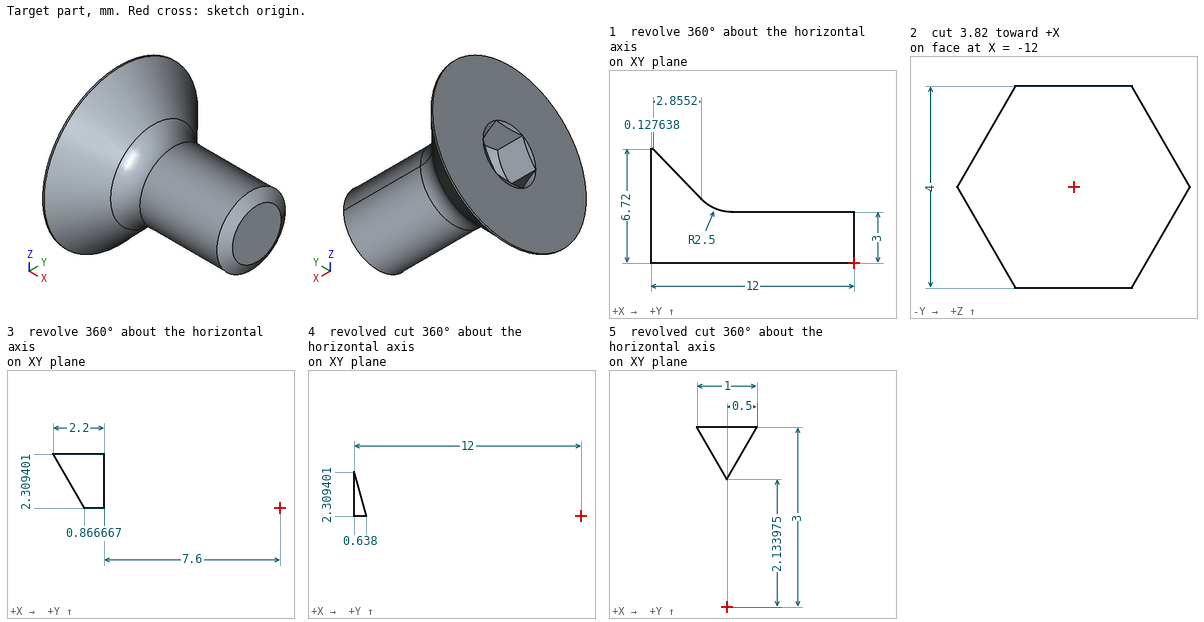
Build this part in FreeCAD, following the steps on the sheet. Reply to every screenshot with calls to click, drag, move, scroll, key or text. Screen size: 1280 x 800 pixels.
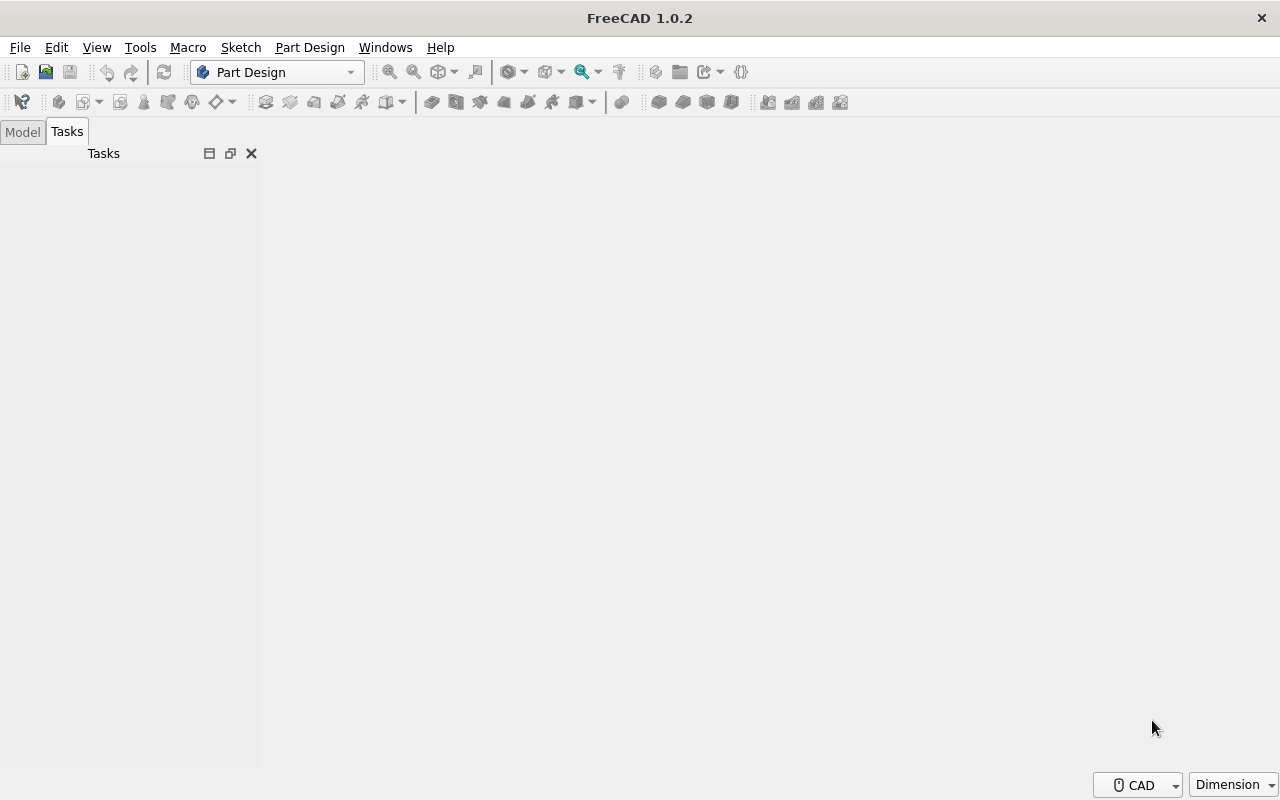
click(22, 72)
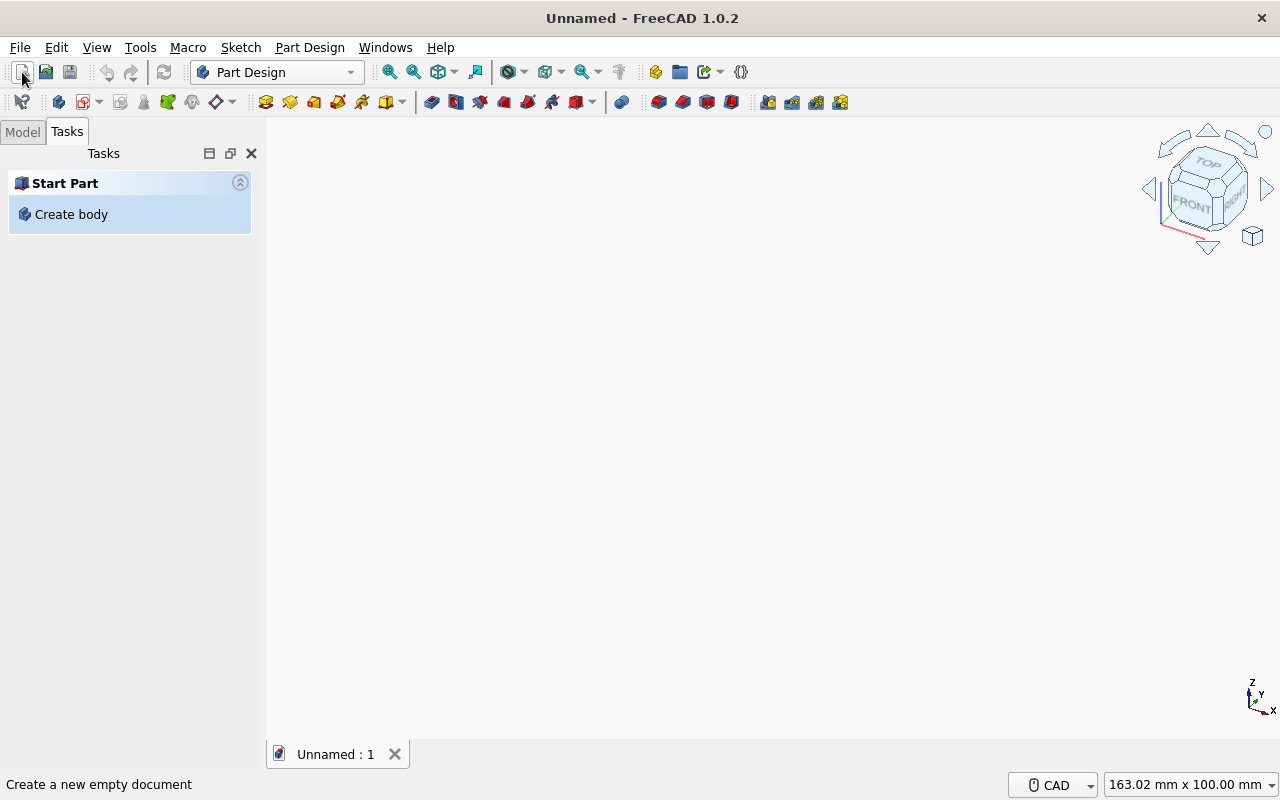
click(84, 102)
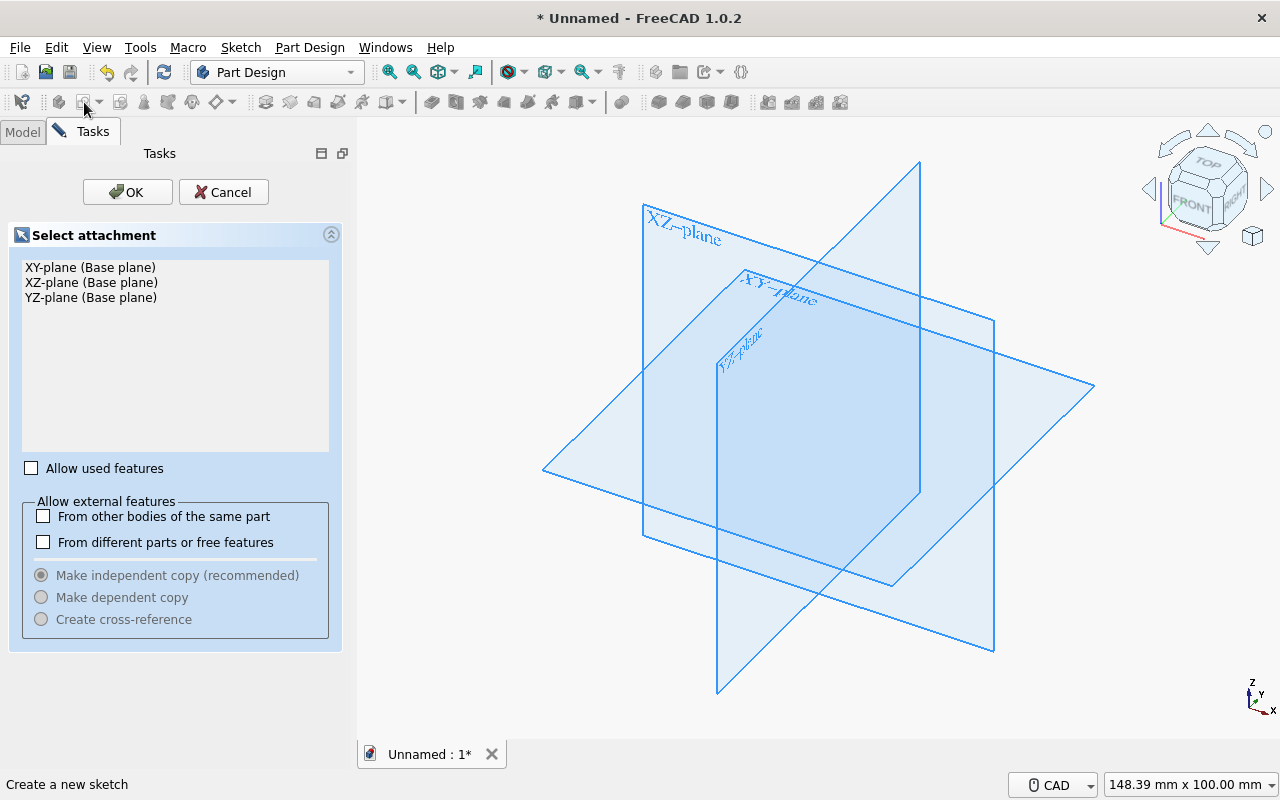
click(82, 268)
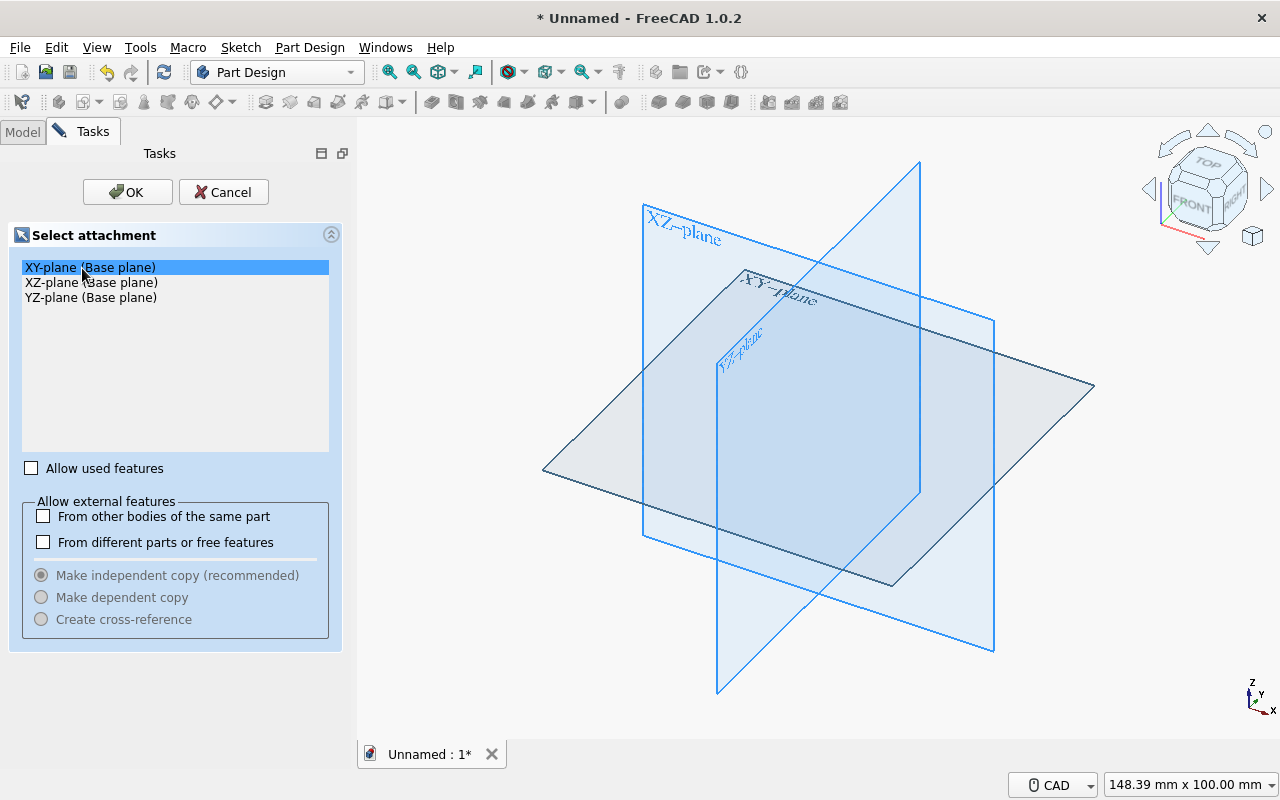
click(128, 192)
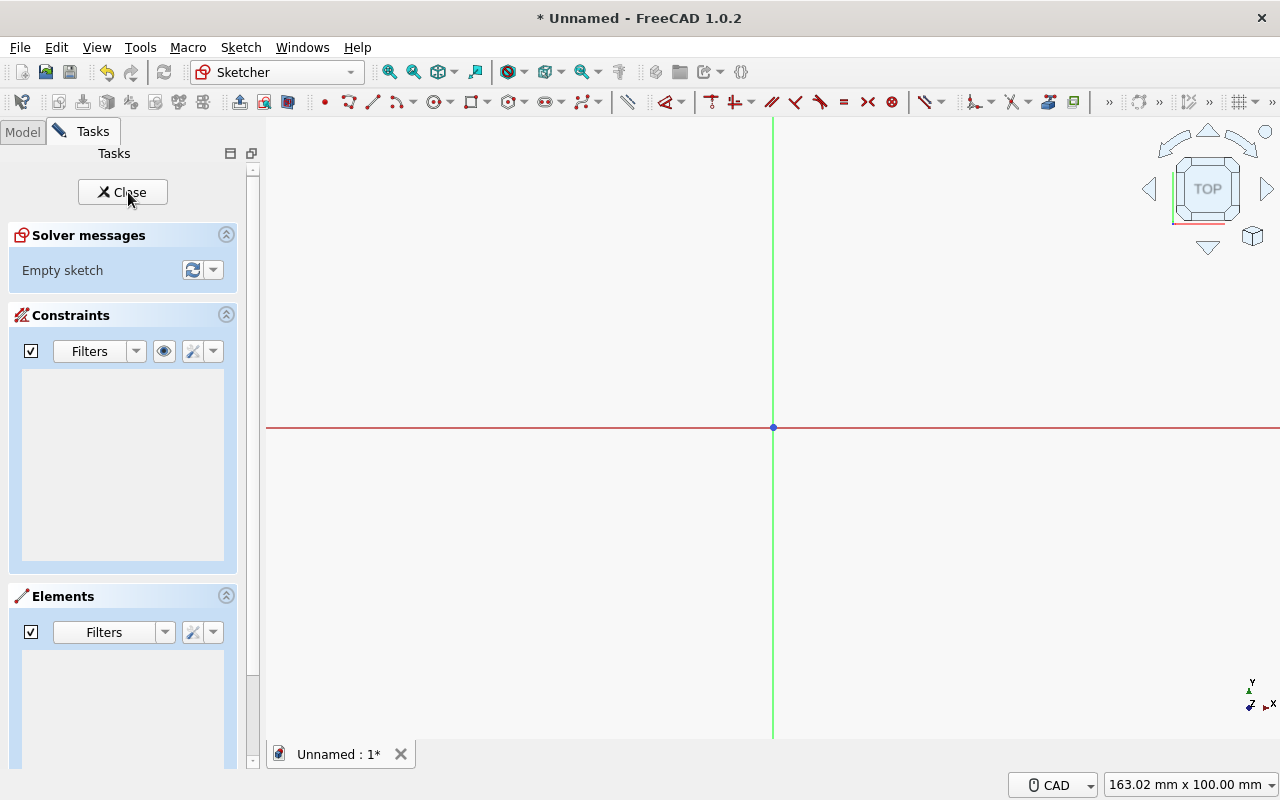
scroll(741, 404, up, 10)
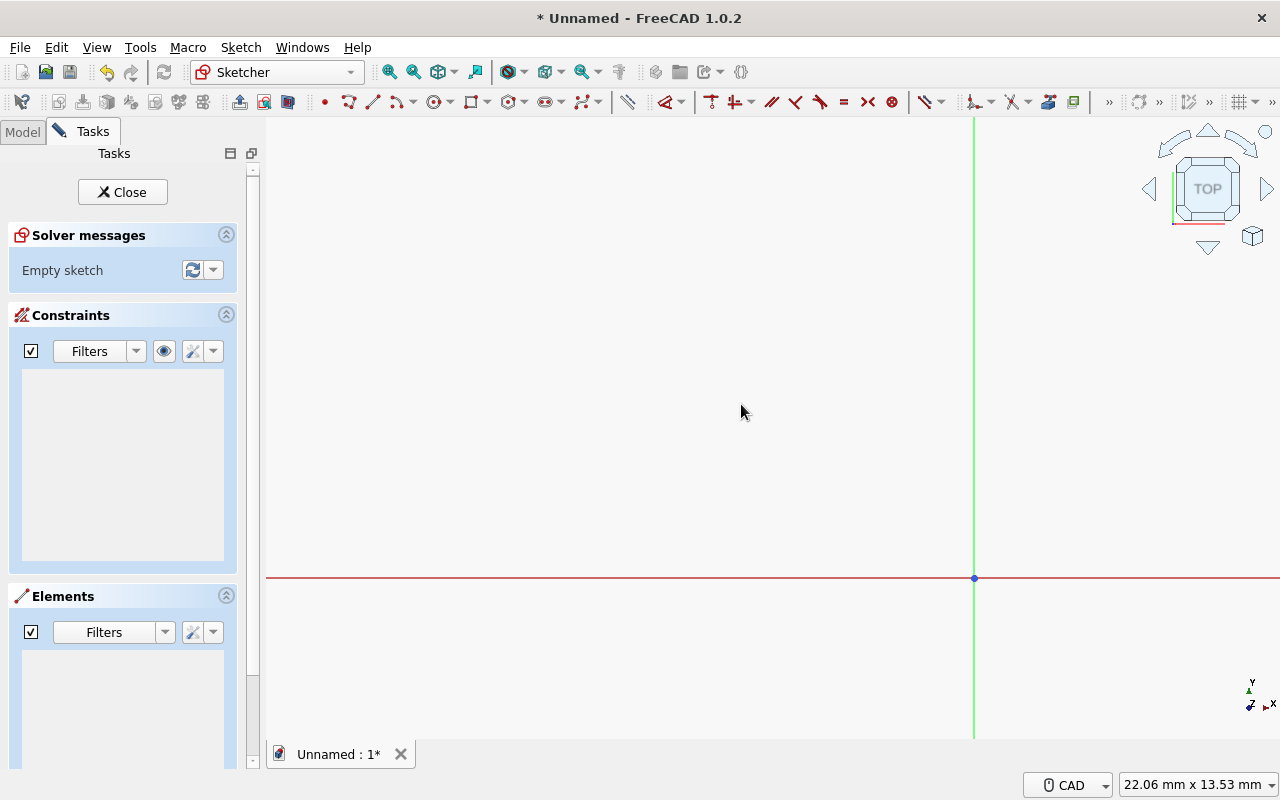
click(350, 102)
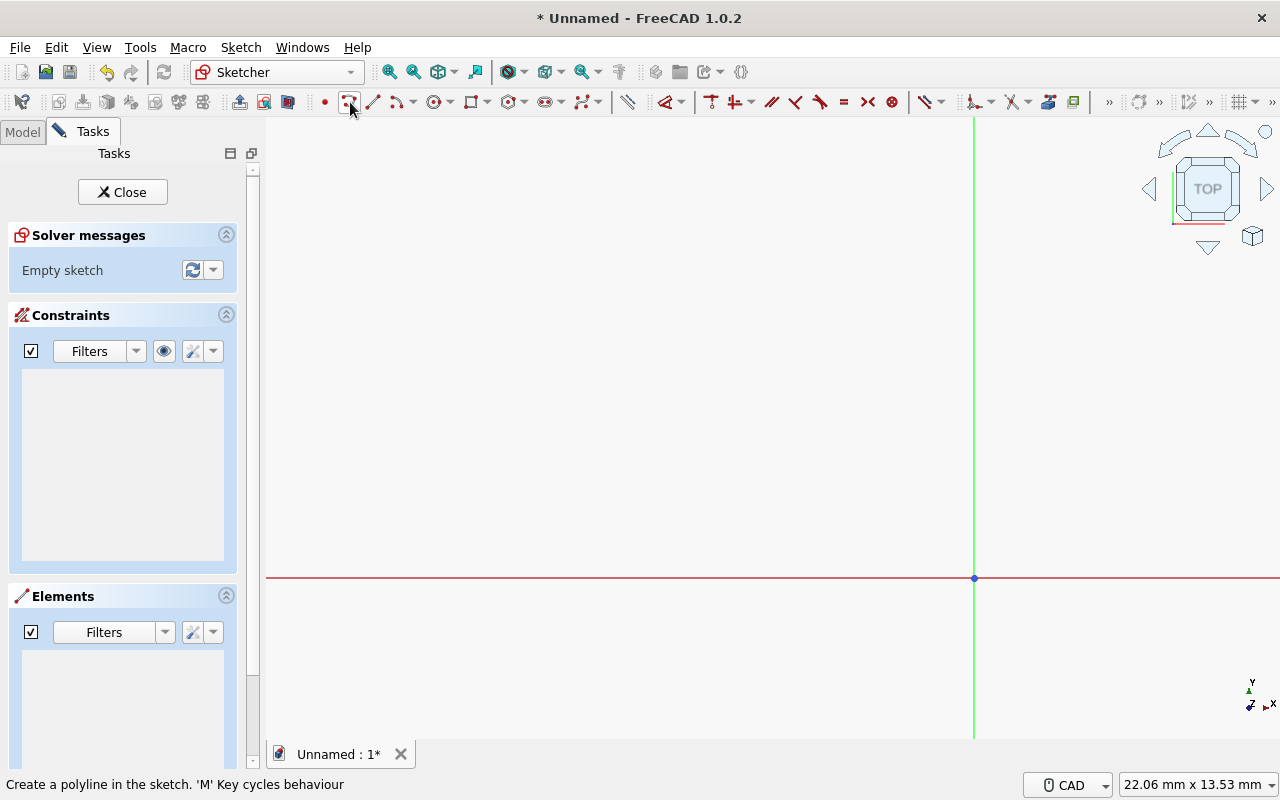
click(560, 405)
click(429, 270)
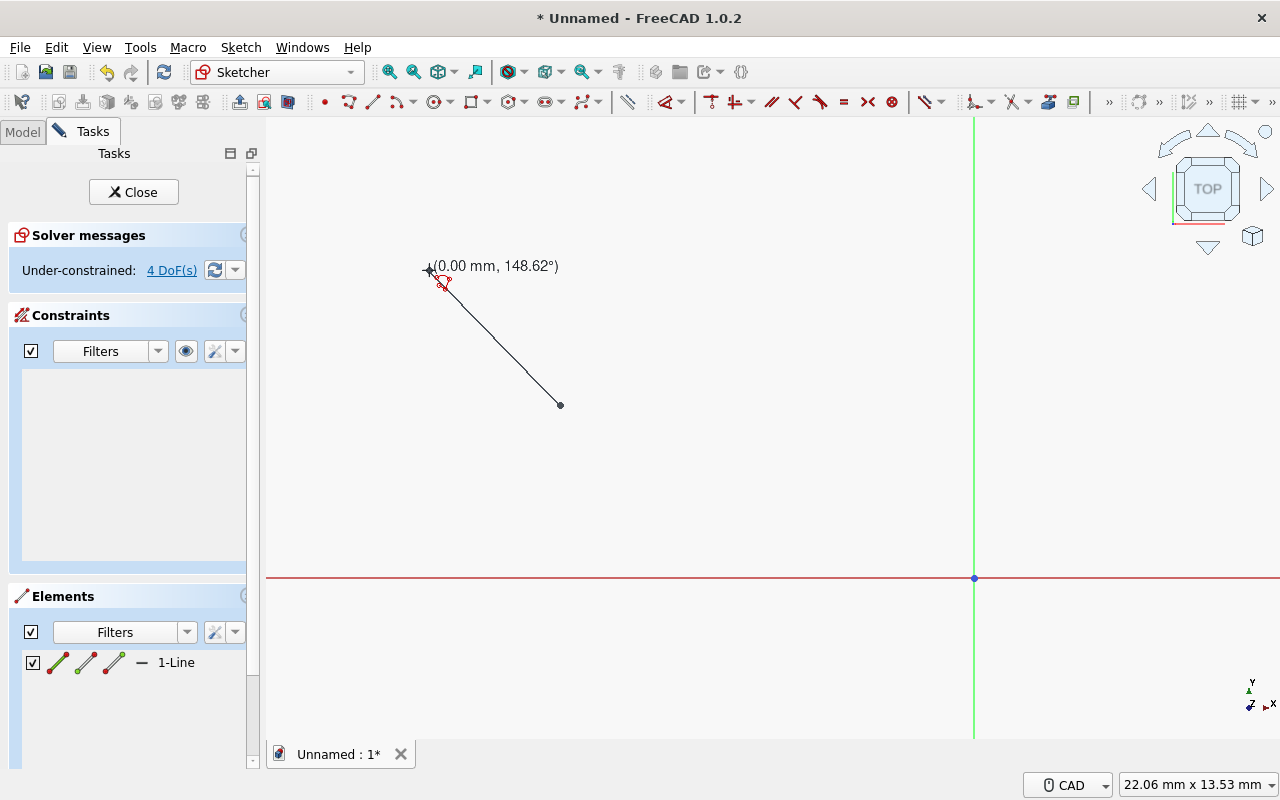
scroll(423, 270, up, 5)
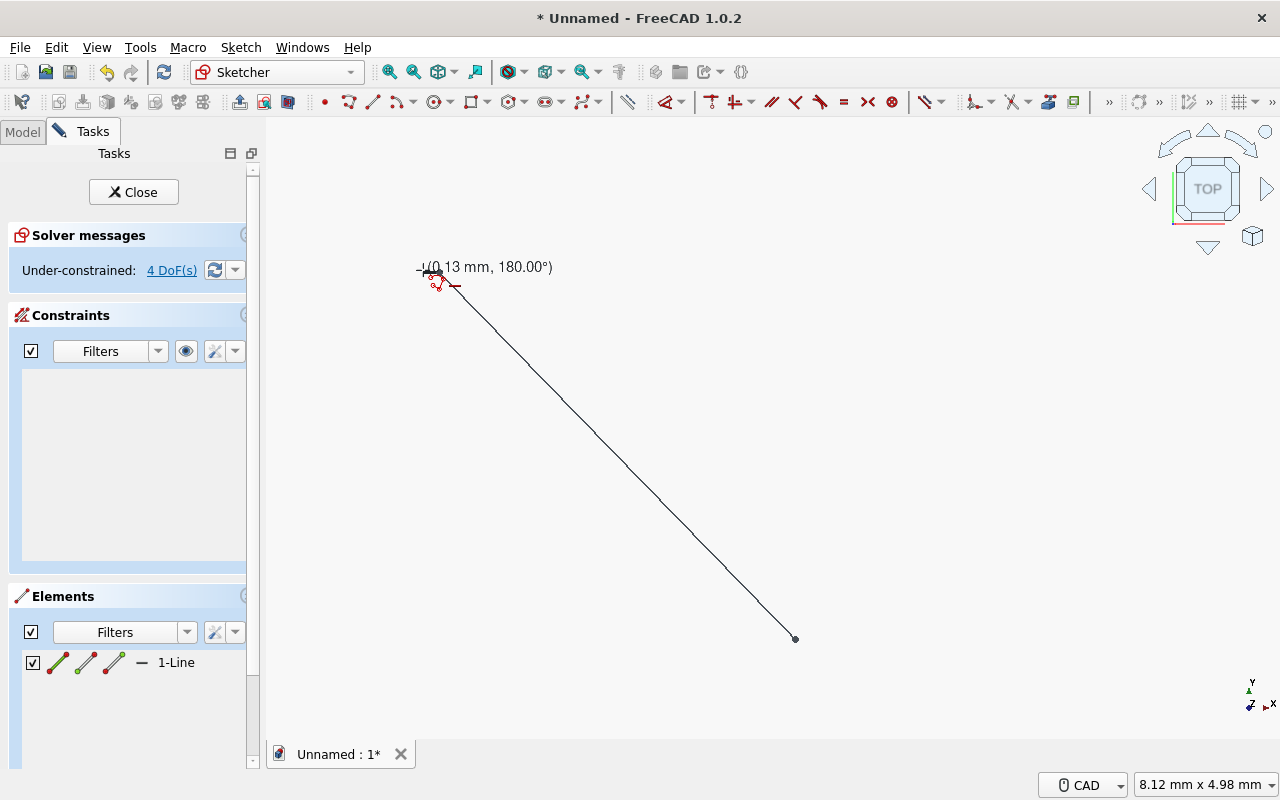
click(423, 270)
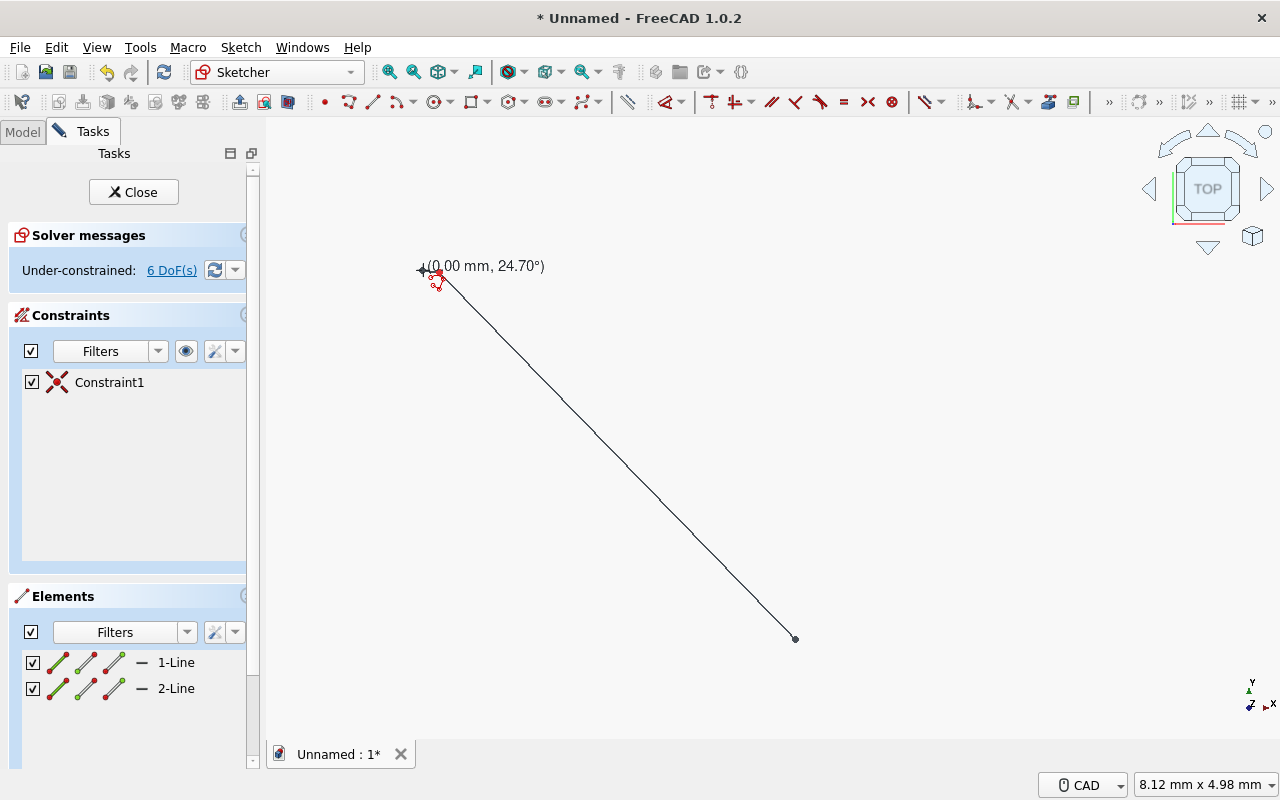
scroll(432, 277, down, 5)